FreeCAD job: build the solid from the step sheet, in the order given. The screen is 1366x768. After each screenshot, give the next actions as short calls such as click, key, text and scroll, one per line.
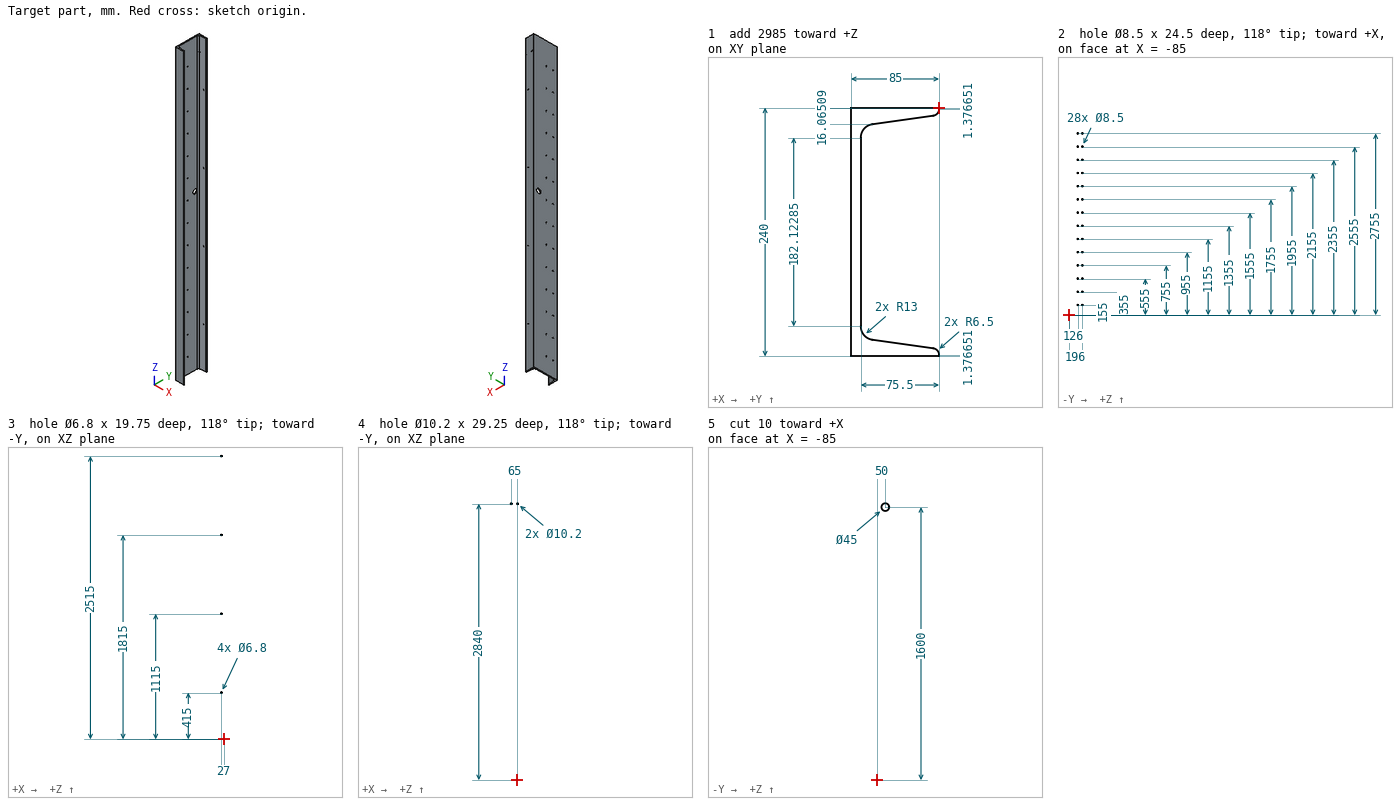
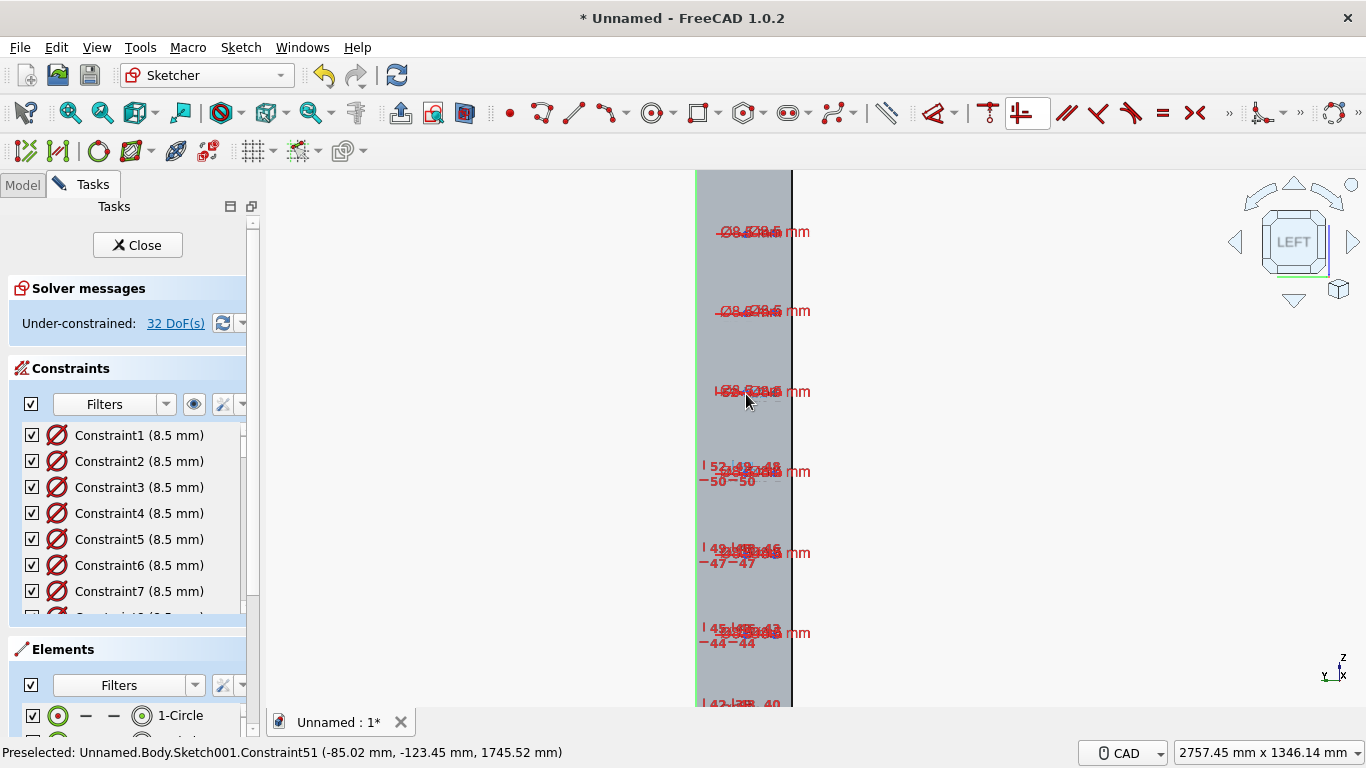
scroll(746, 393, up, 4)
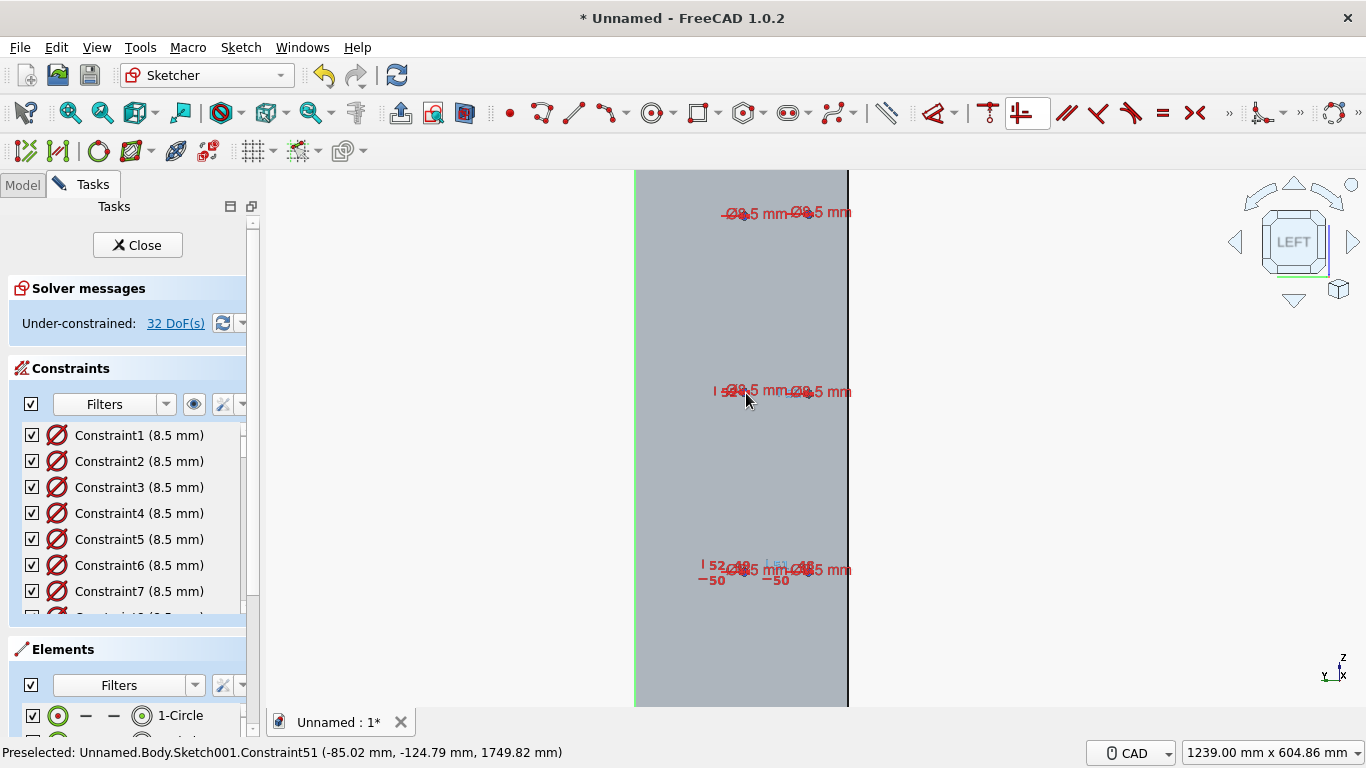
click(744, 392)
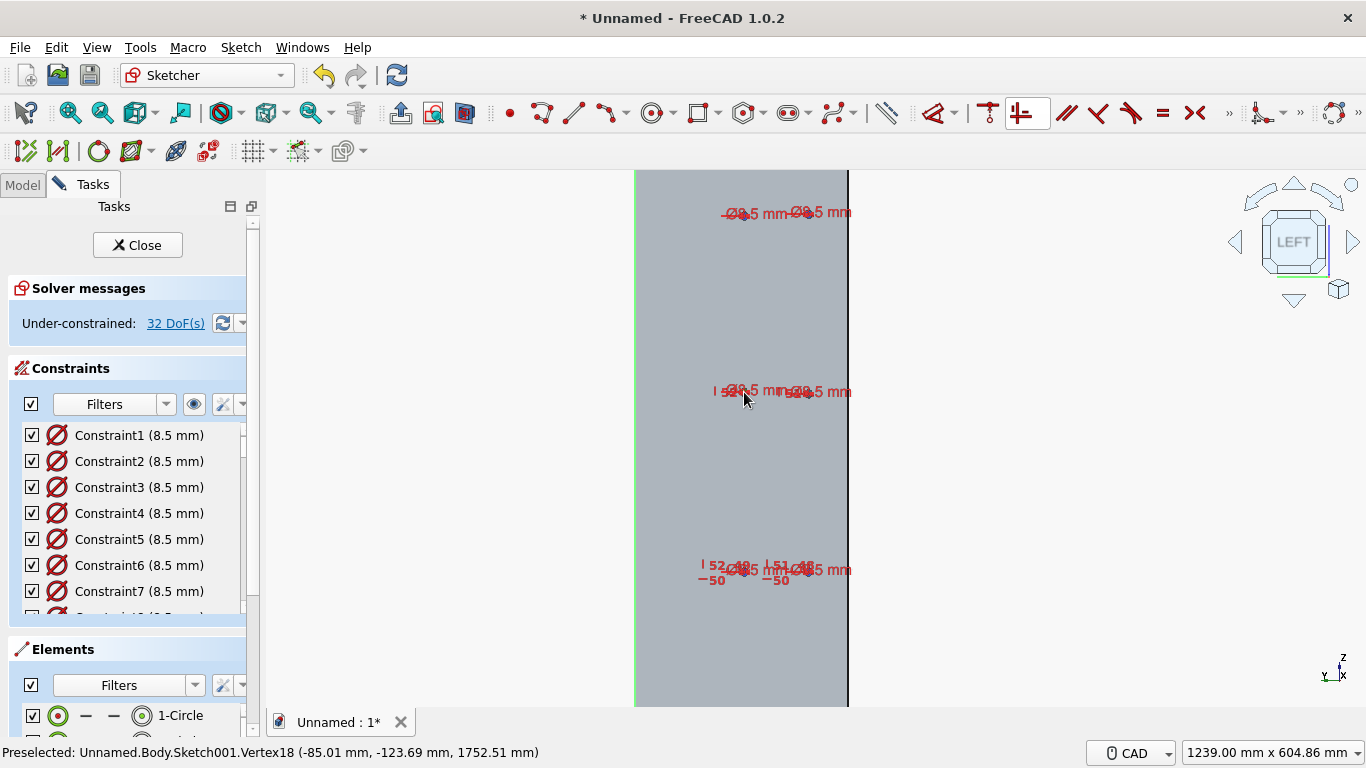
click(1044, 114)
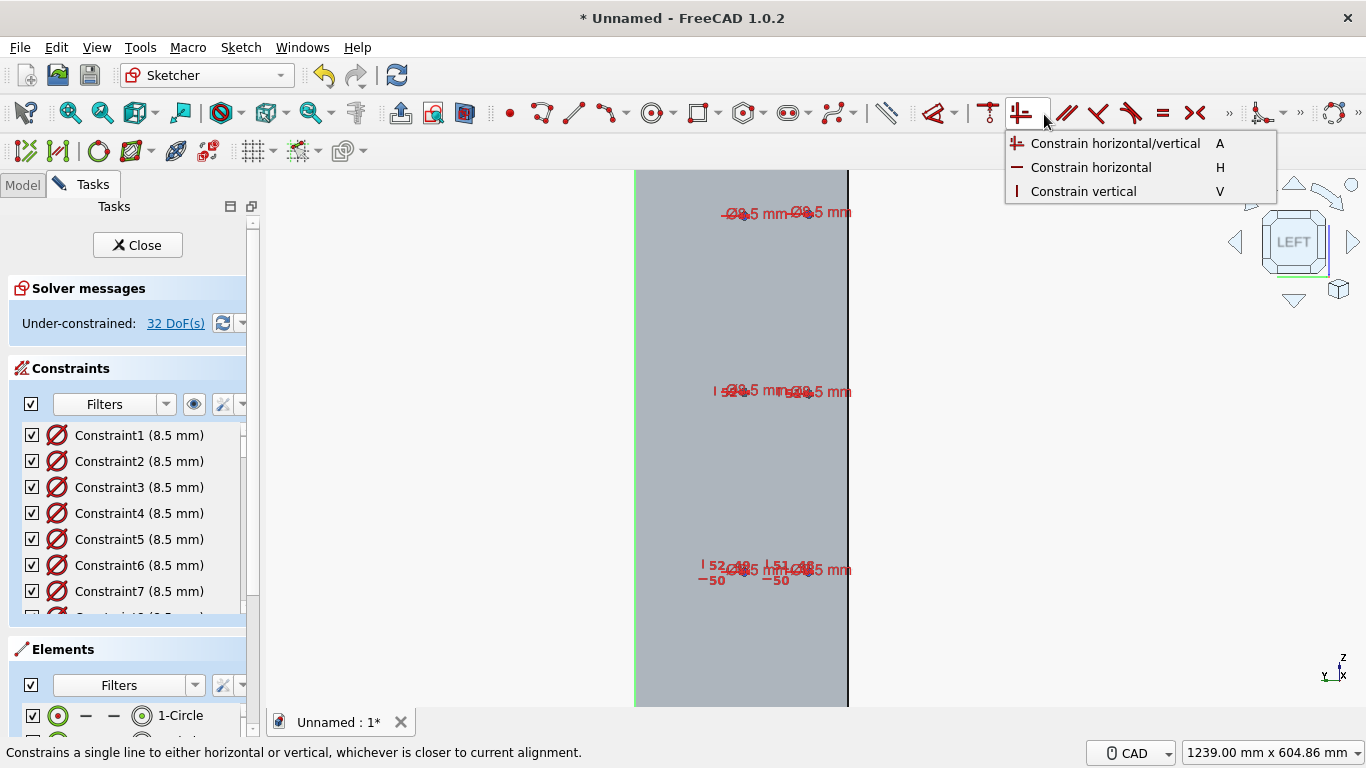
click(1141, 167)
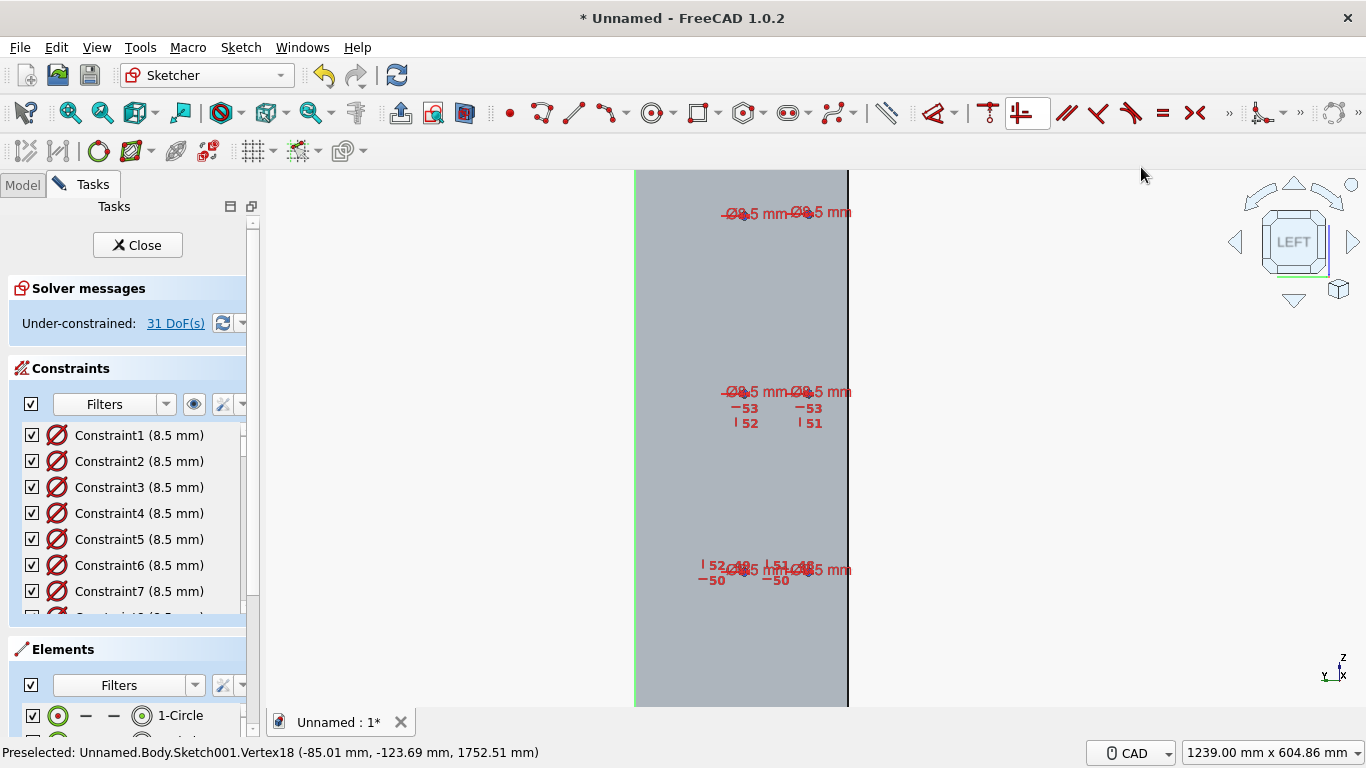
scroll(751, 394, down, 10)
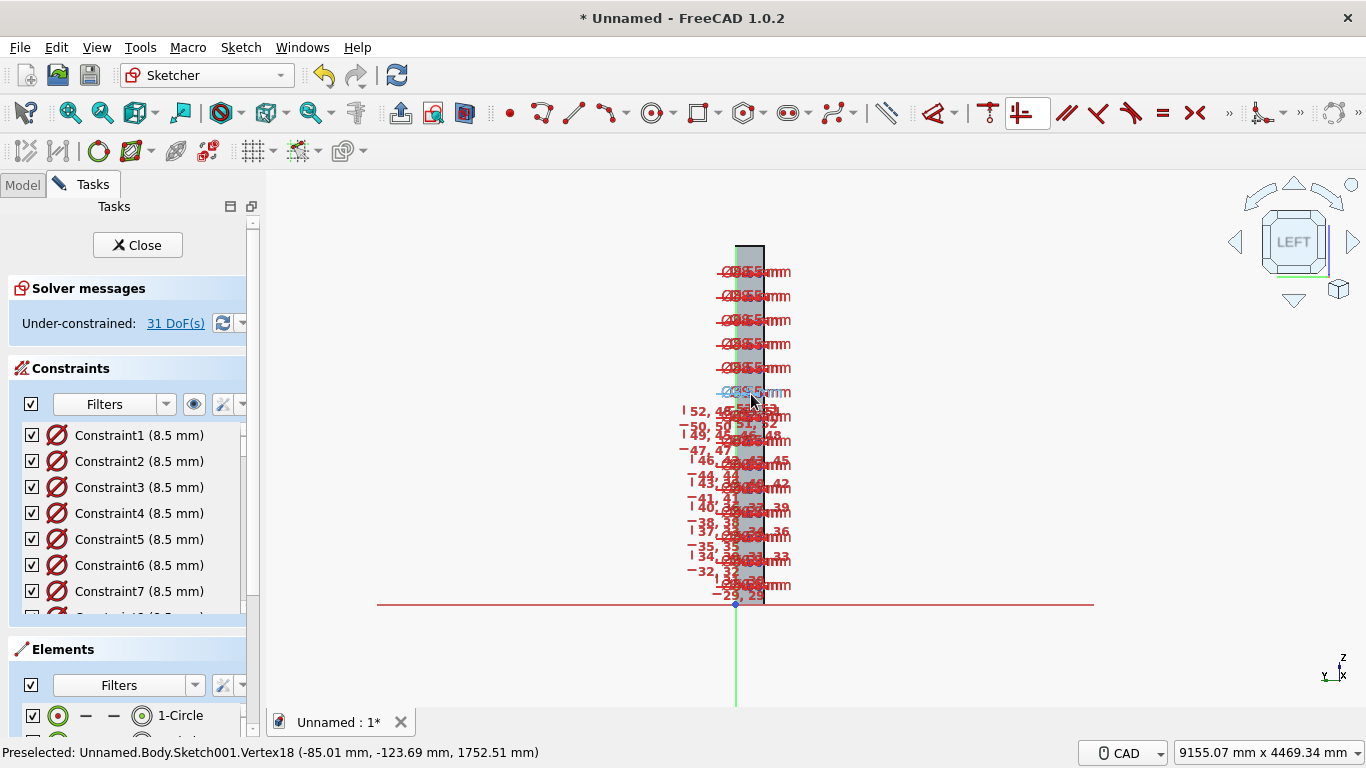
scroll(751, 394, up, 2)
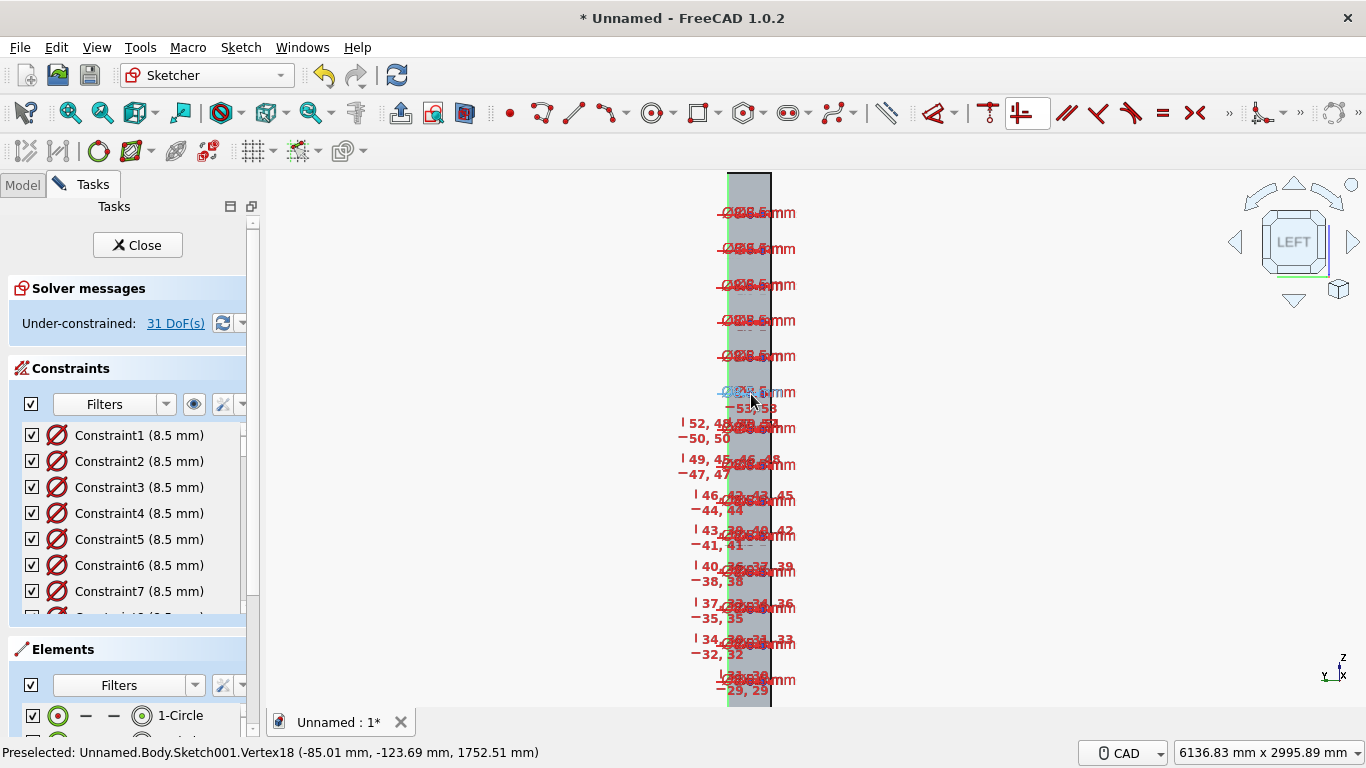
click(750, 394)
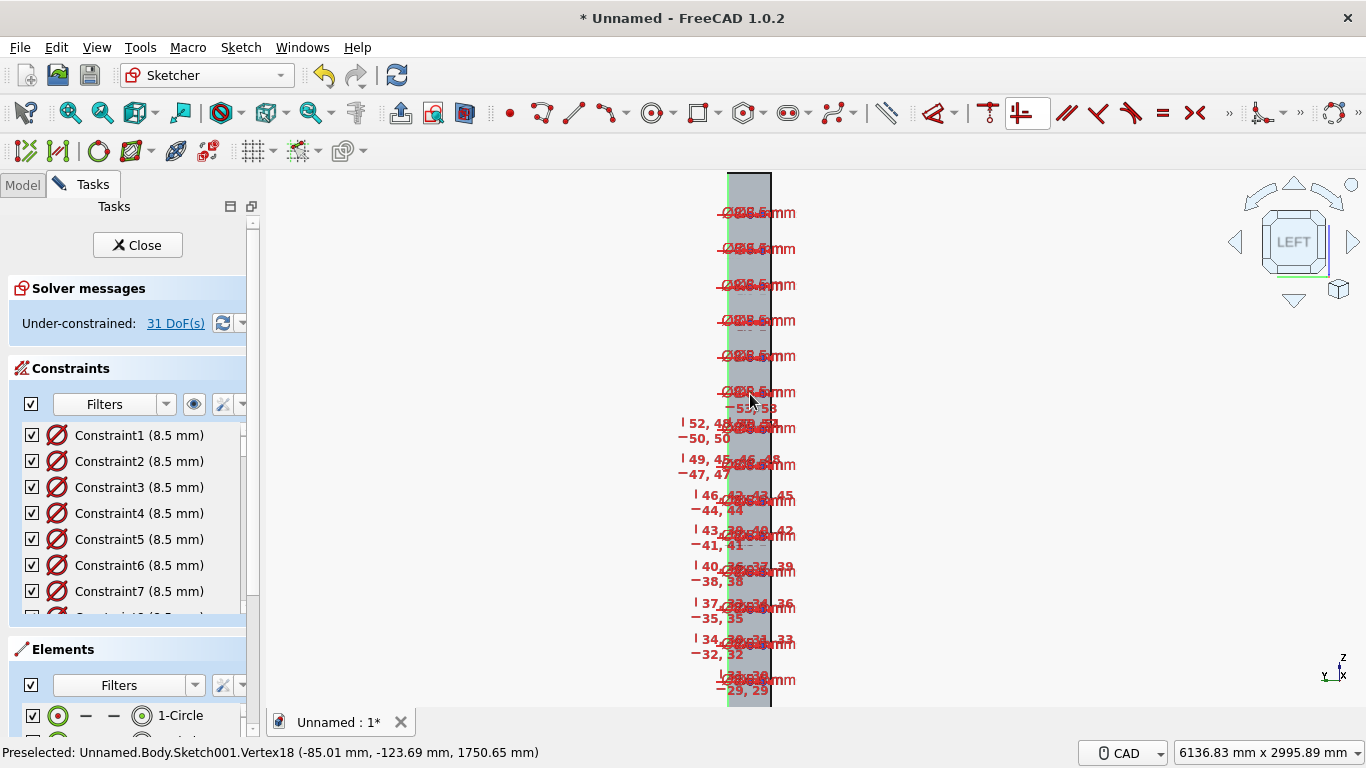
click(750, 358)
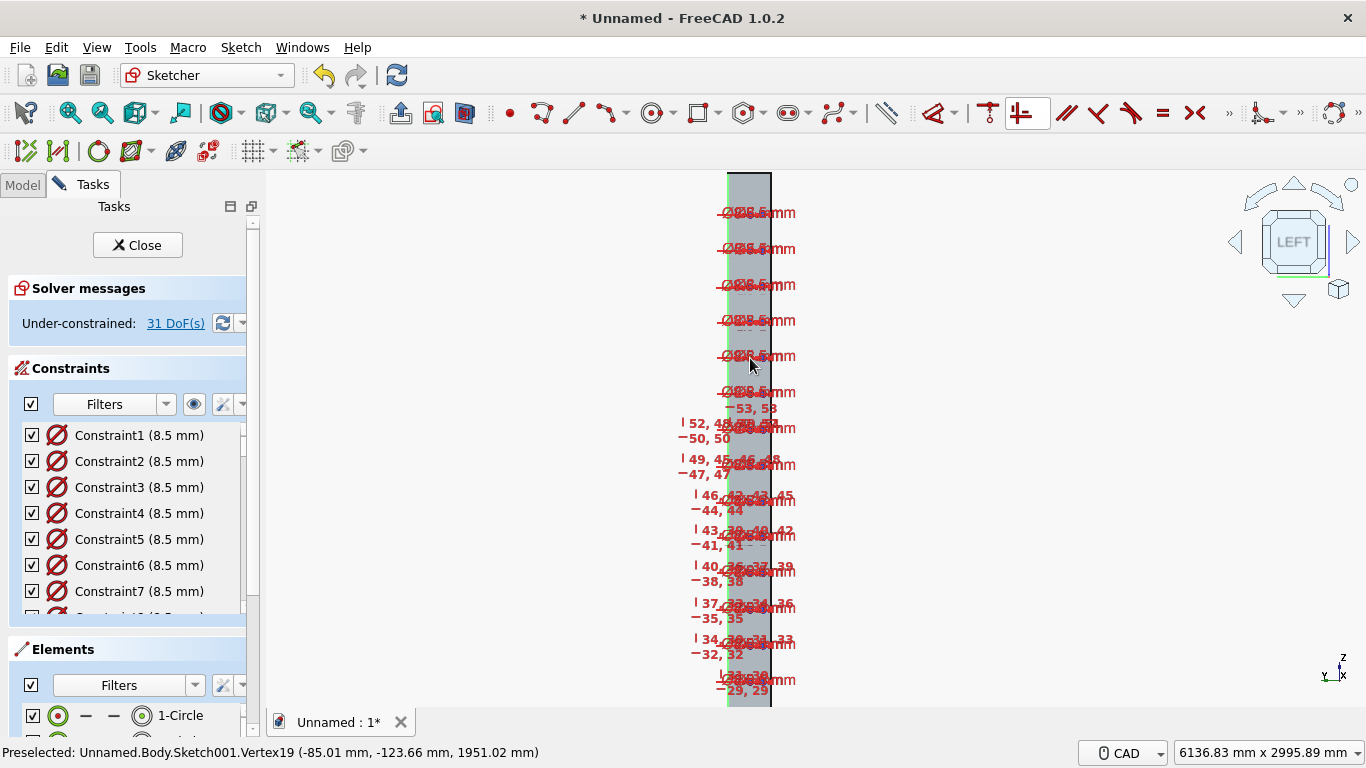
click(1044, 114)